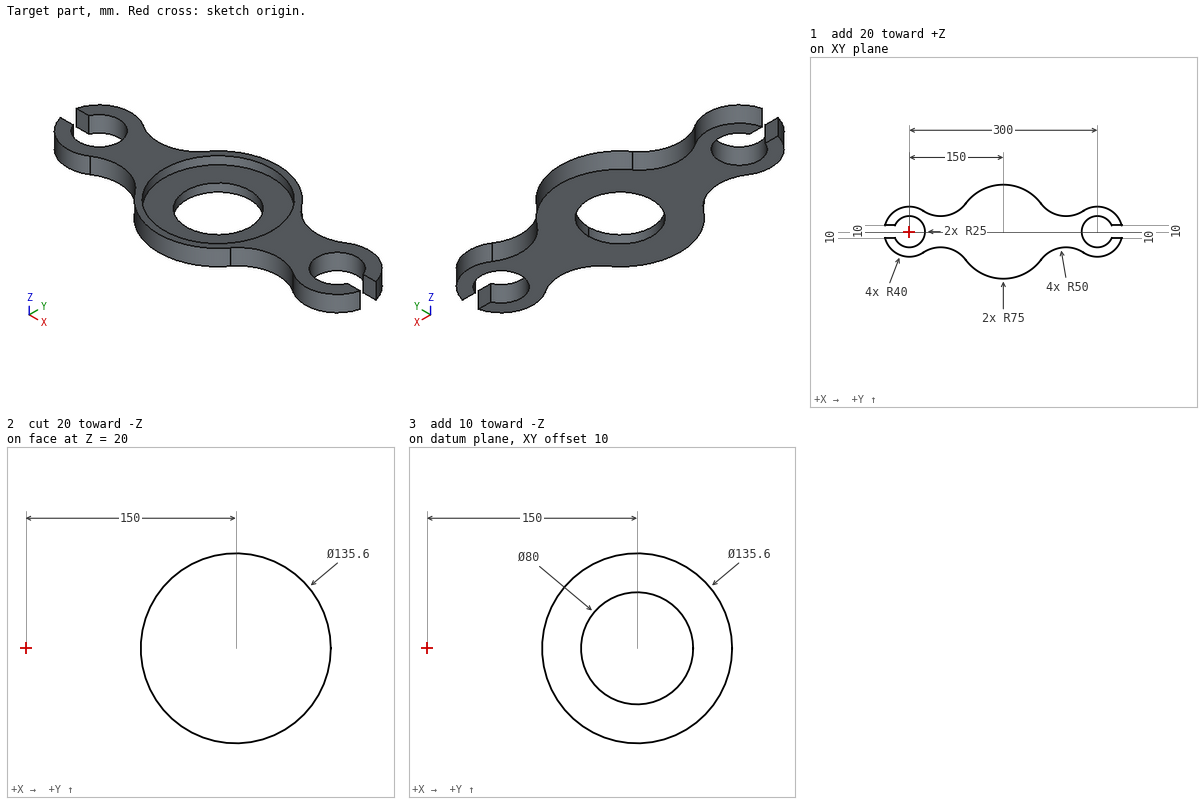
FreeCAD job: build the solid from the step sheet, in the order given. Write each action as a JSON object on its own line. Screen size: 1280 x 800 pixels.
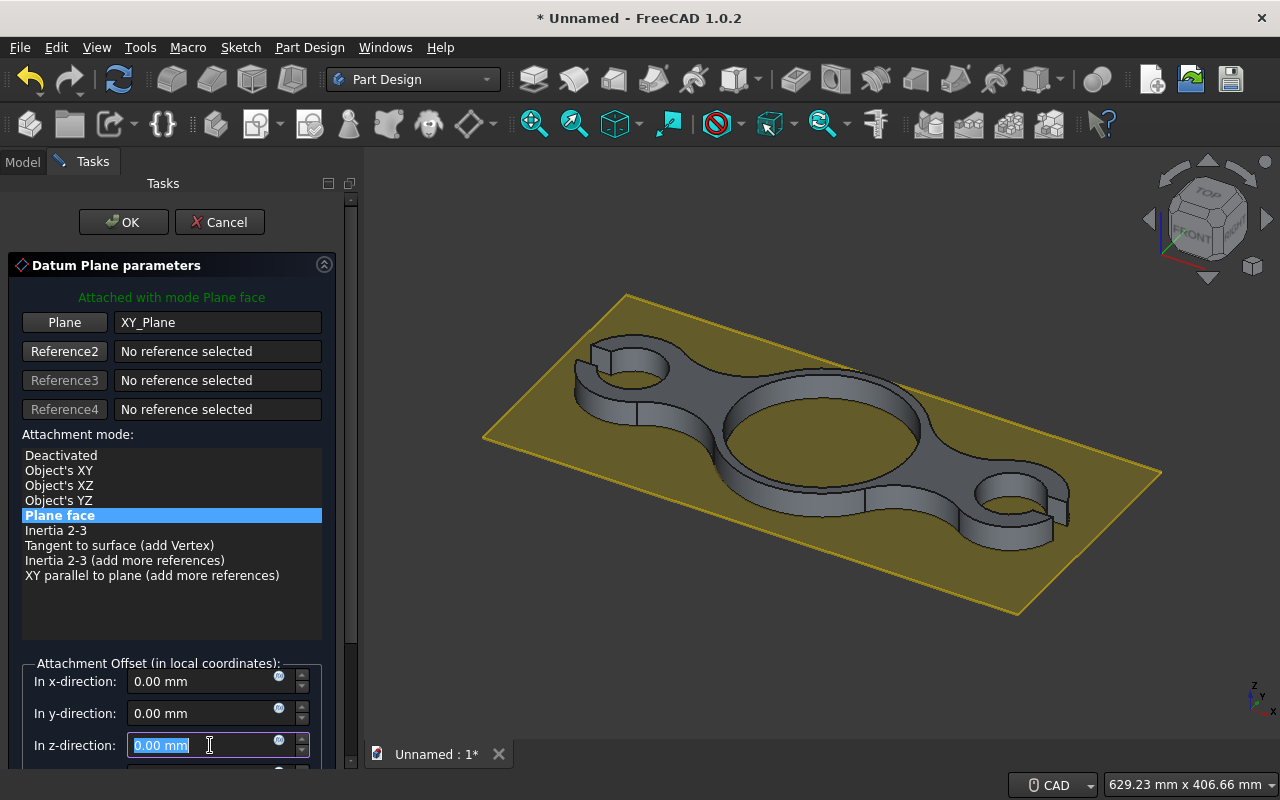
{"action": "type", "text": "10"}
{"action": "key", "text": "Tab"}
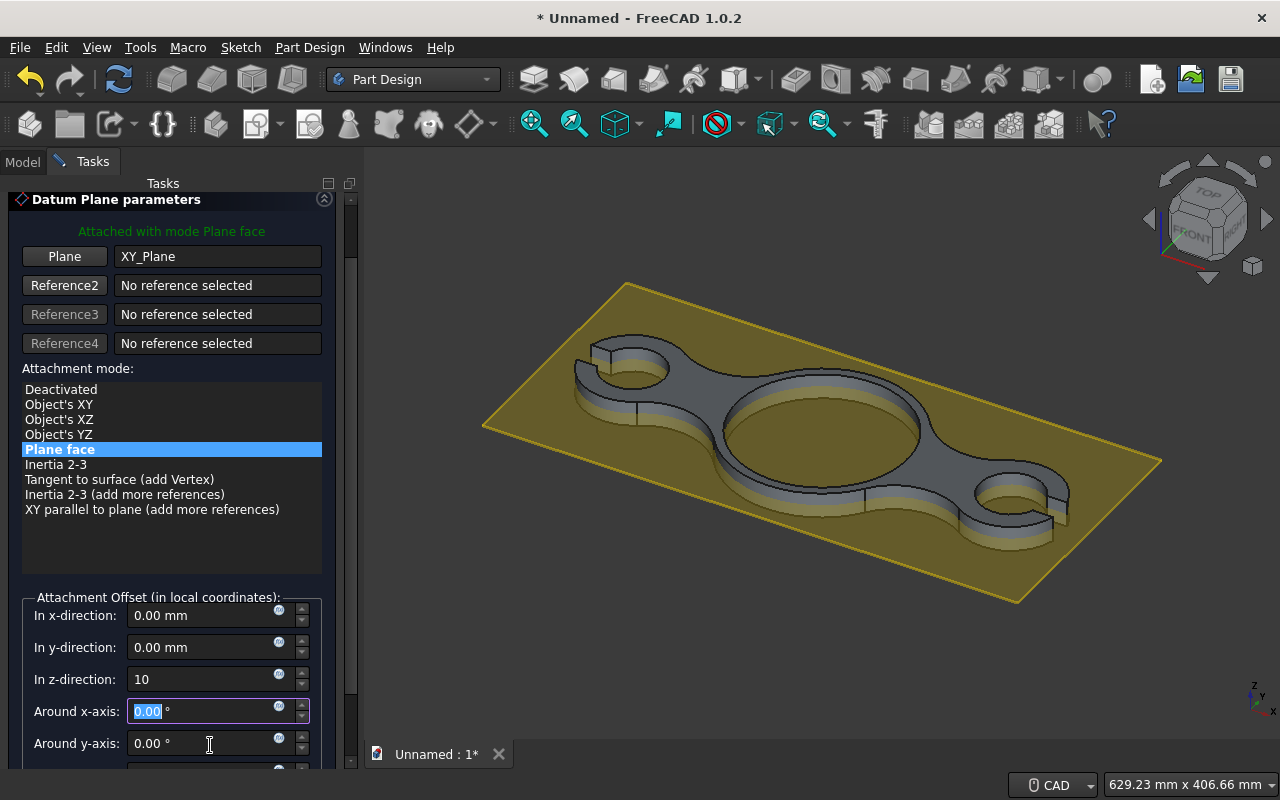
{"action": "scroll", "coordinate": [351, 480], "scroll_direction": "up", "scroll_amount": 2}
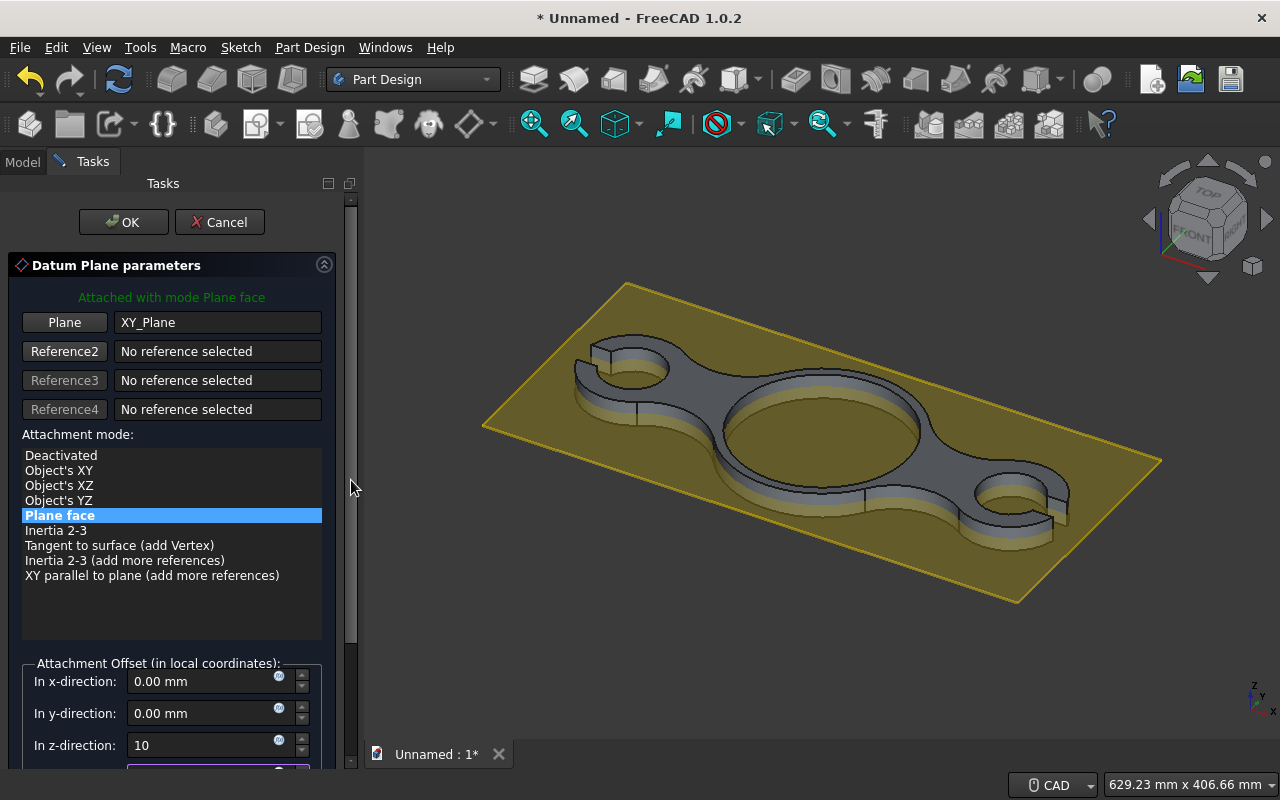
{"action": "left_click", "coordinate": [124, 222]}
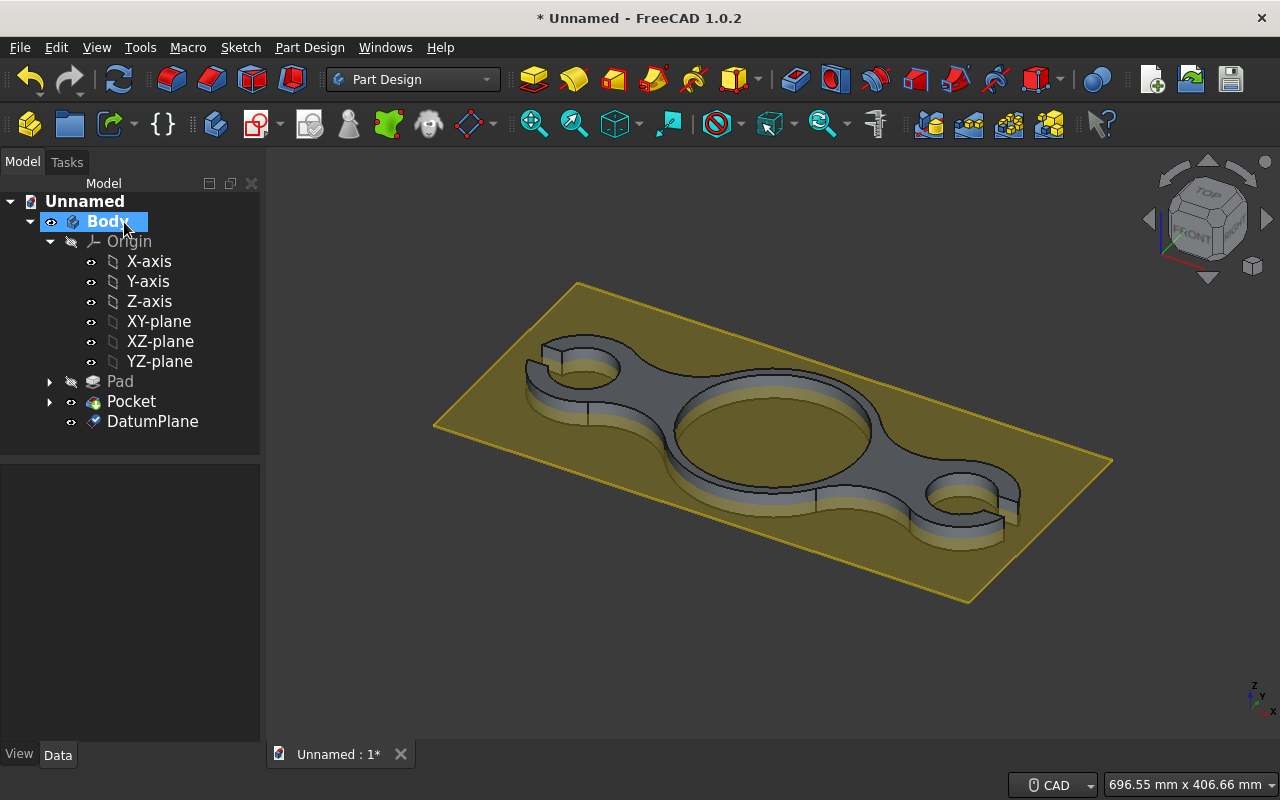
{"action": "left_click", "coordinate": [116, 422]}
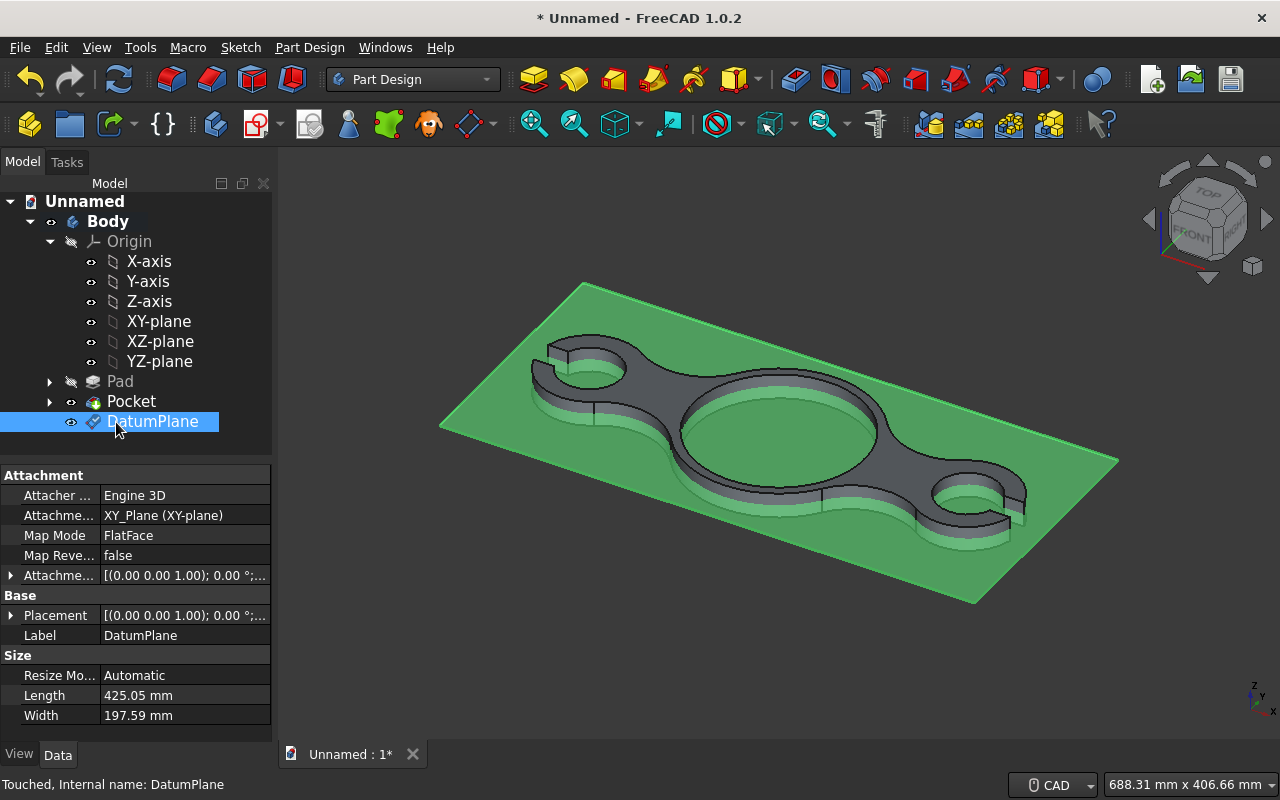
{"action": "left_click", "coordinate": [256, 124]}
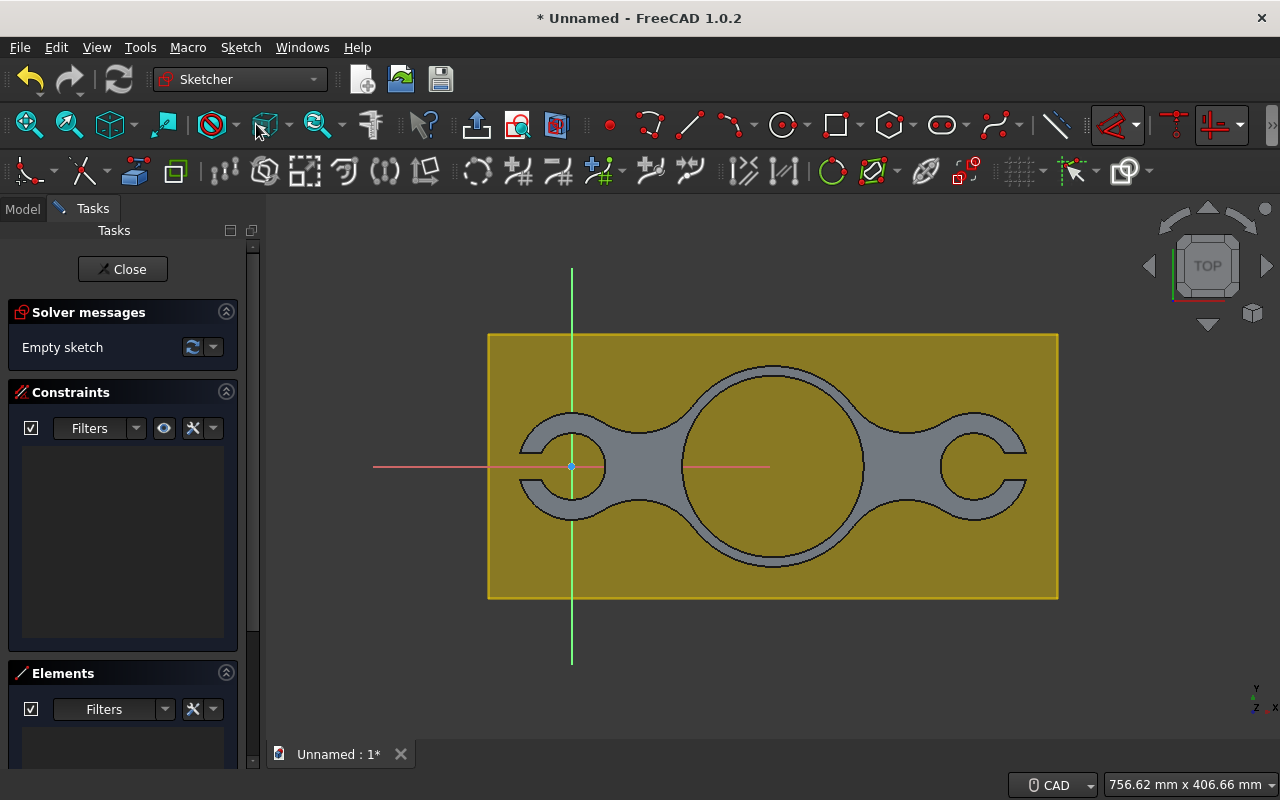
{"action": "left_click", "coordinate": [558, 126]}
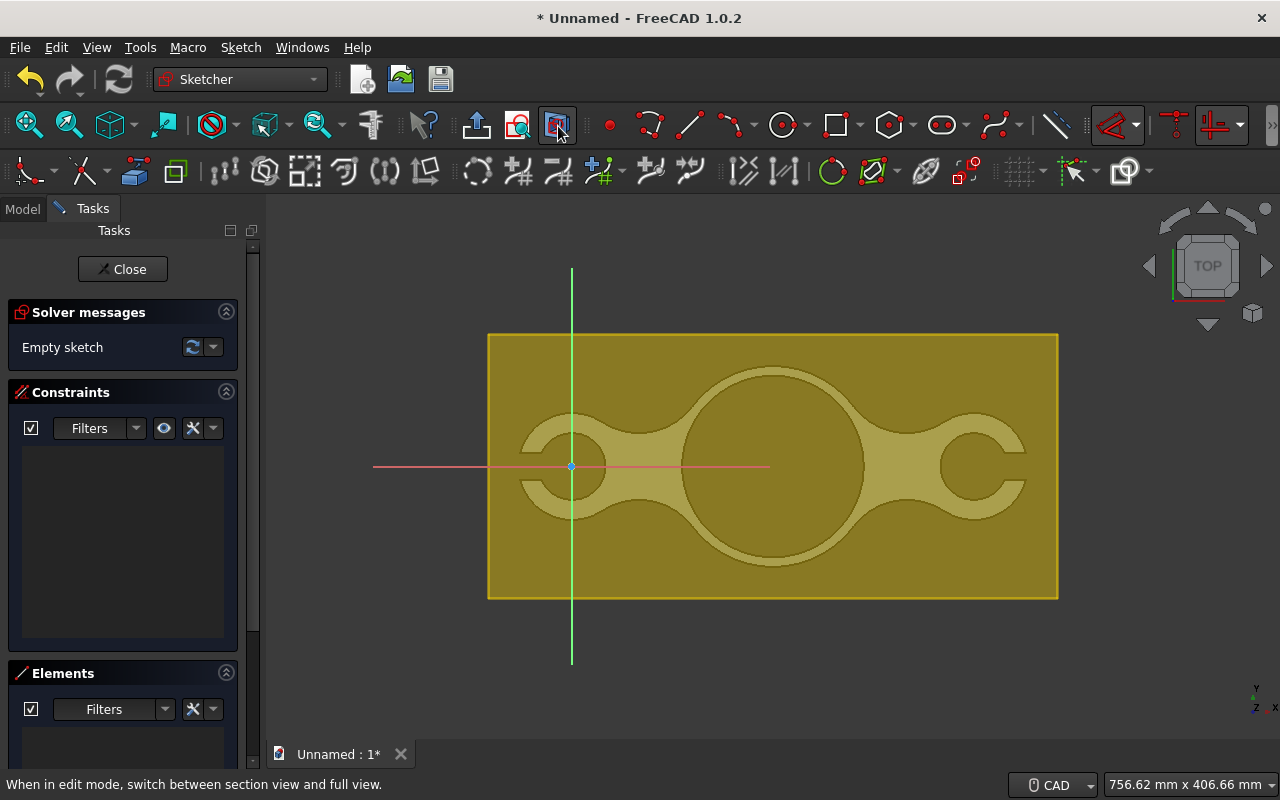
{"action": "scroll", "coordinate": [734, 466], "scroll_direction": "up", "scroll_amount": 3}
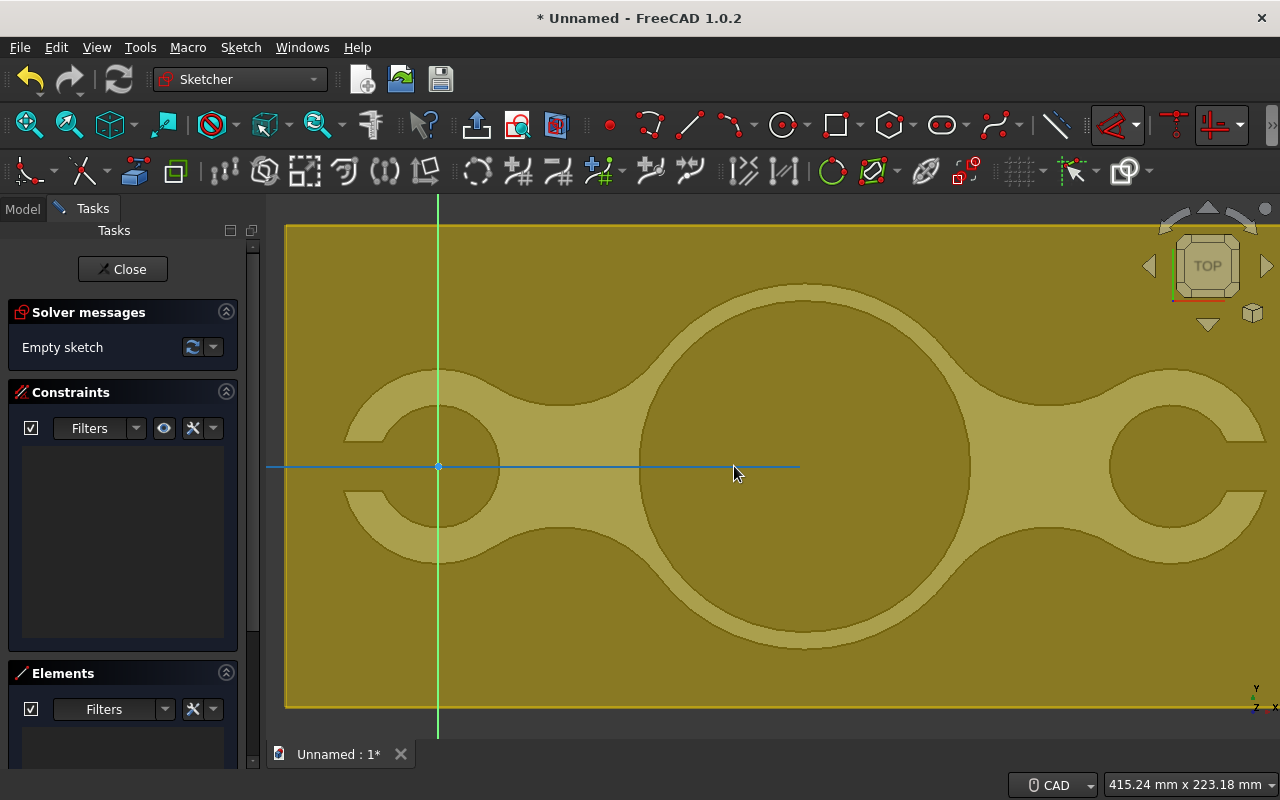
{"action": "left_click", "coordinate": [784, 126]}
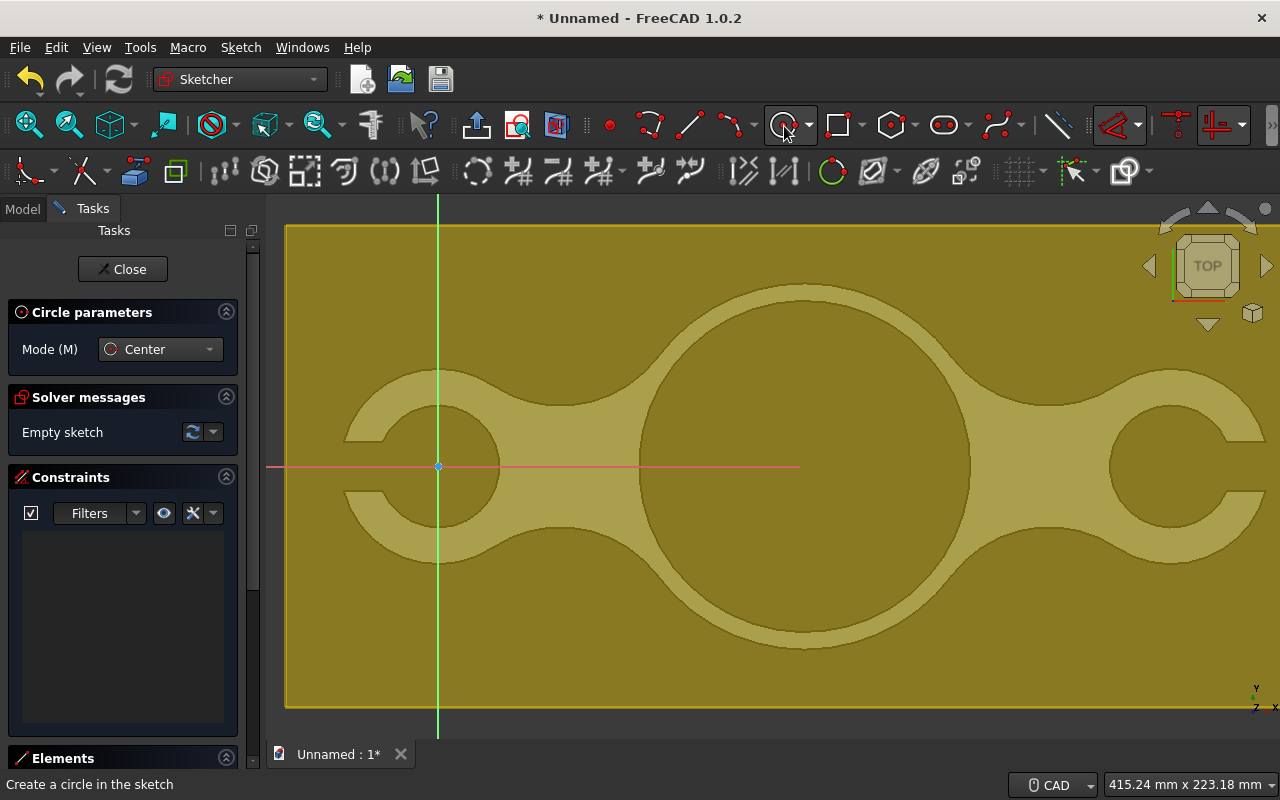
{"action": "left_click", "coordinate": [805, 466]}
{"action": "mouse_move", "coordinate": [922, 349]}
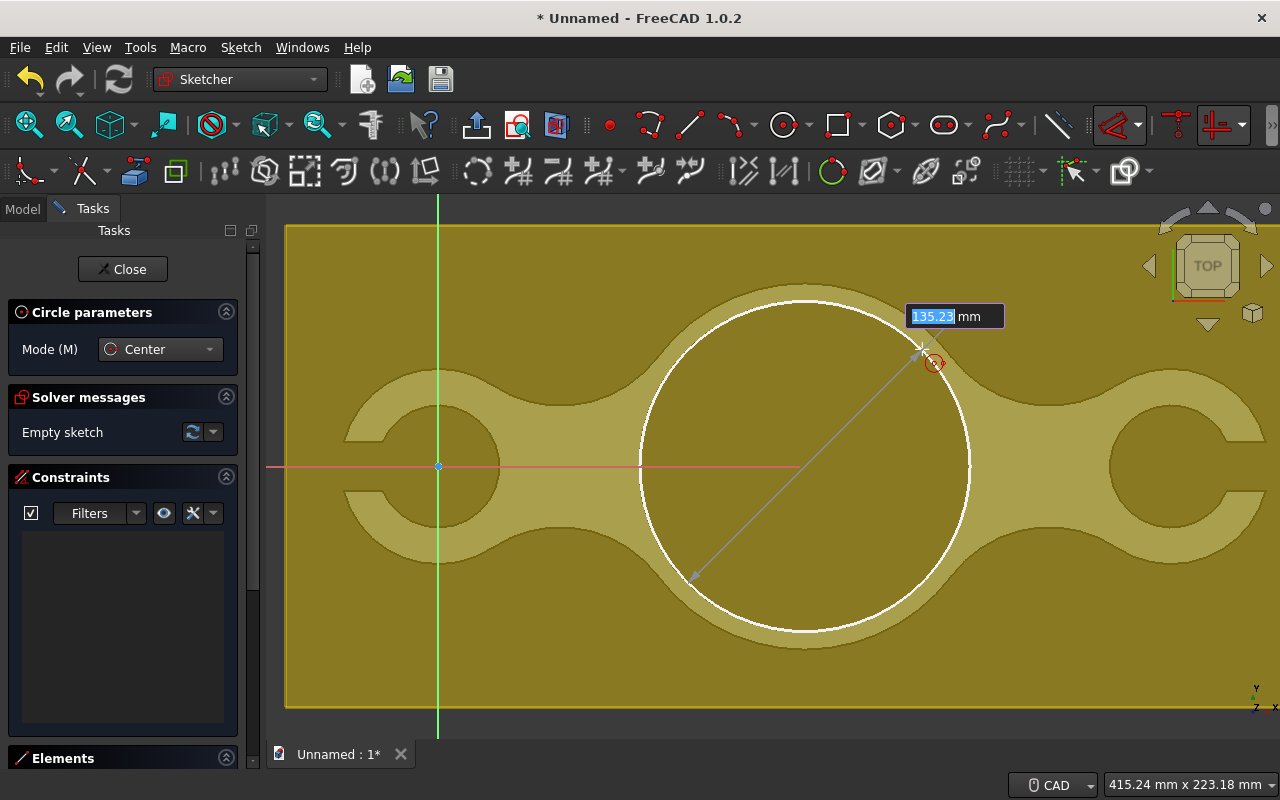
{"action": "type", "text": "135.6"}
{"action": "key", "text": "Return"}